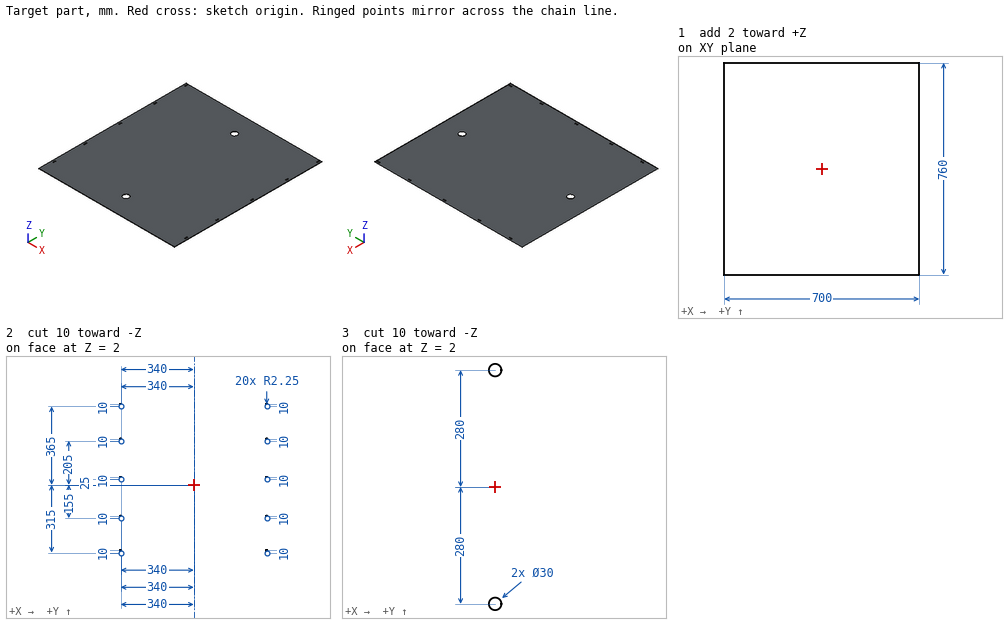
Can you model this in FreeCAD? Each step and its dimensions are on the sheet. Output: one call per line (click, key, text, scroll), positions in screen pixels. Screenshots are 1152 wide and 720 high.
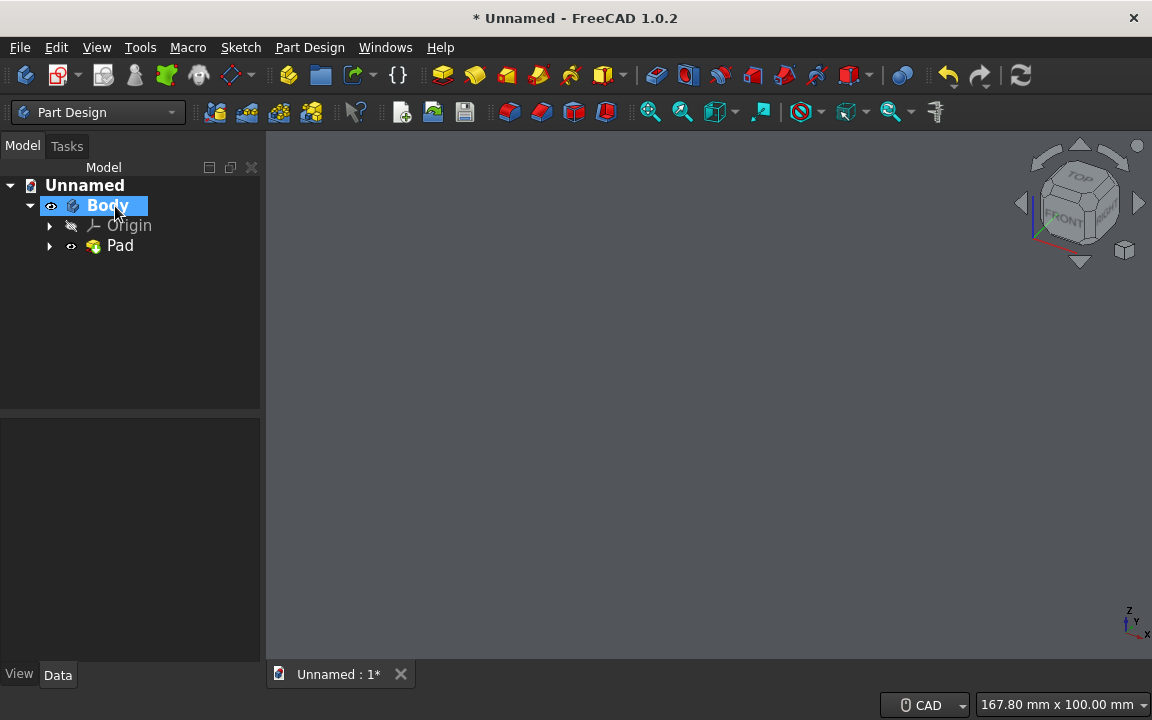
click(652, 112)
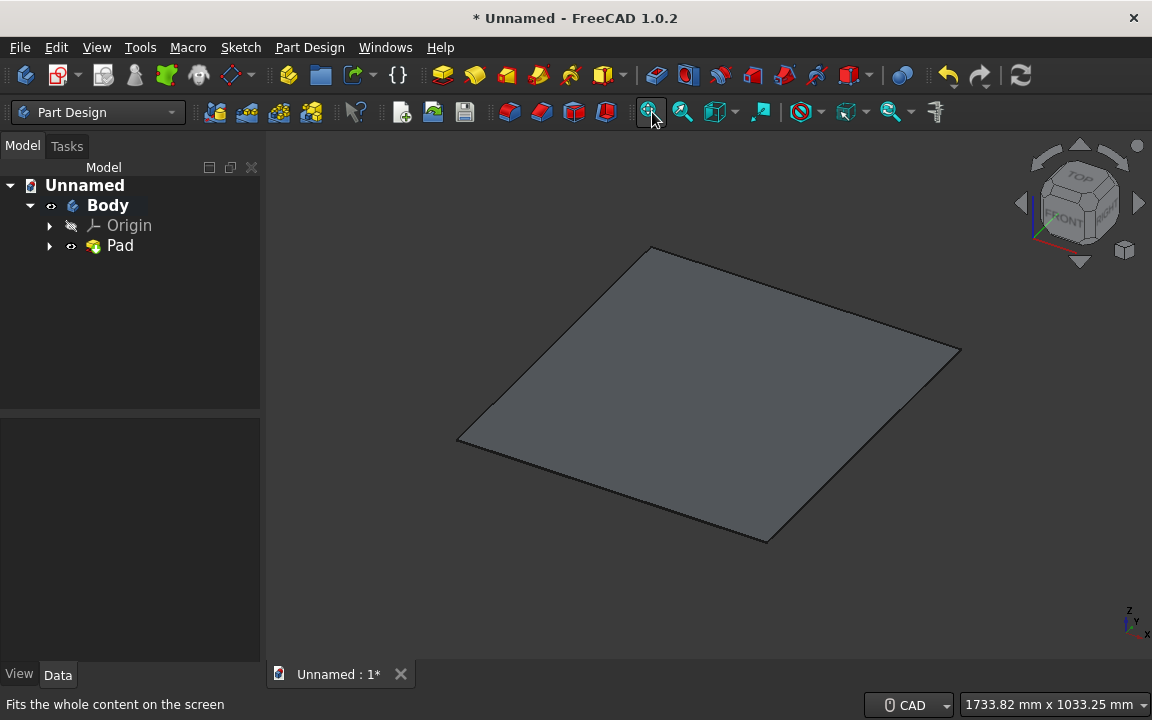
click(709, 394)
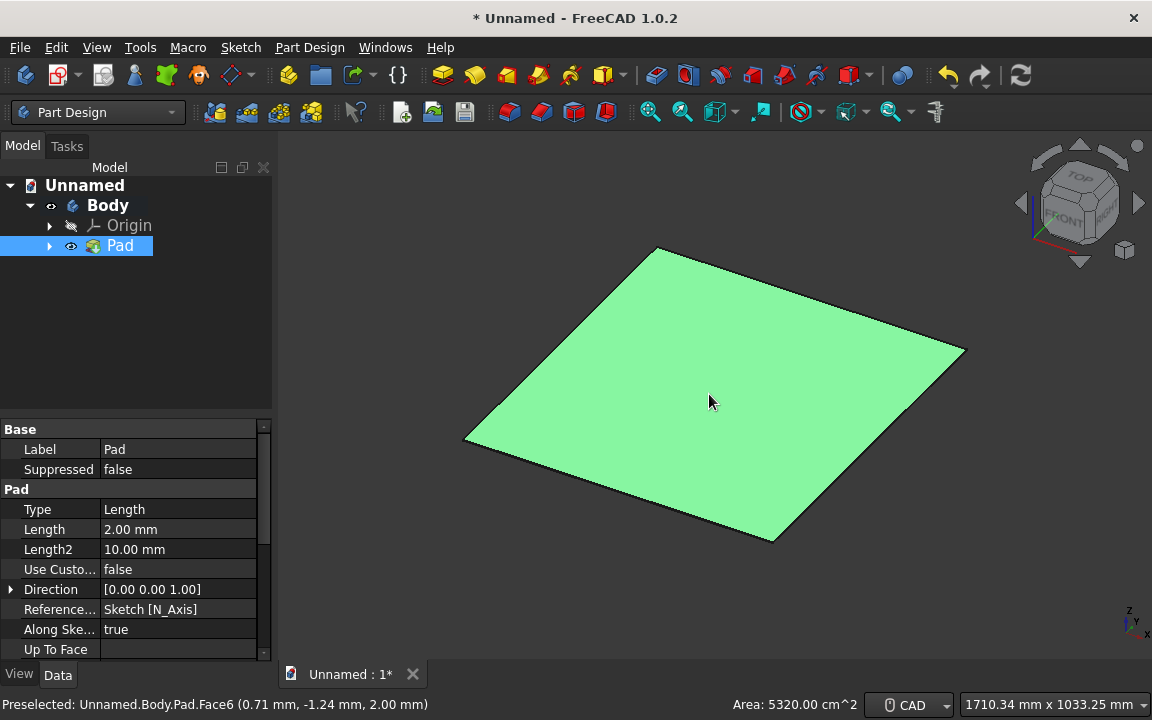
click(58, 76)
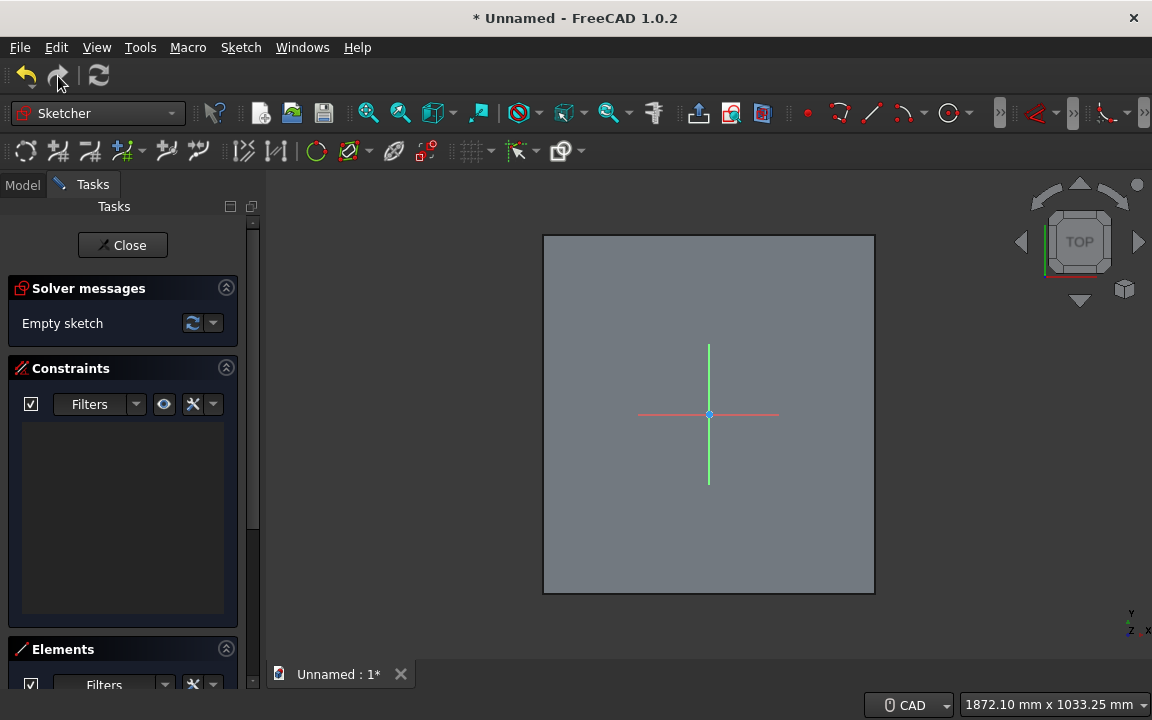
key(g)
key(s)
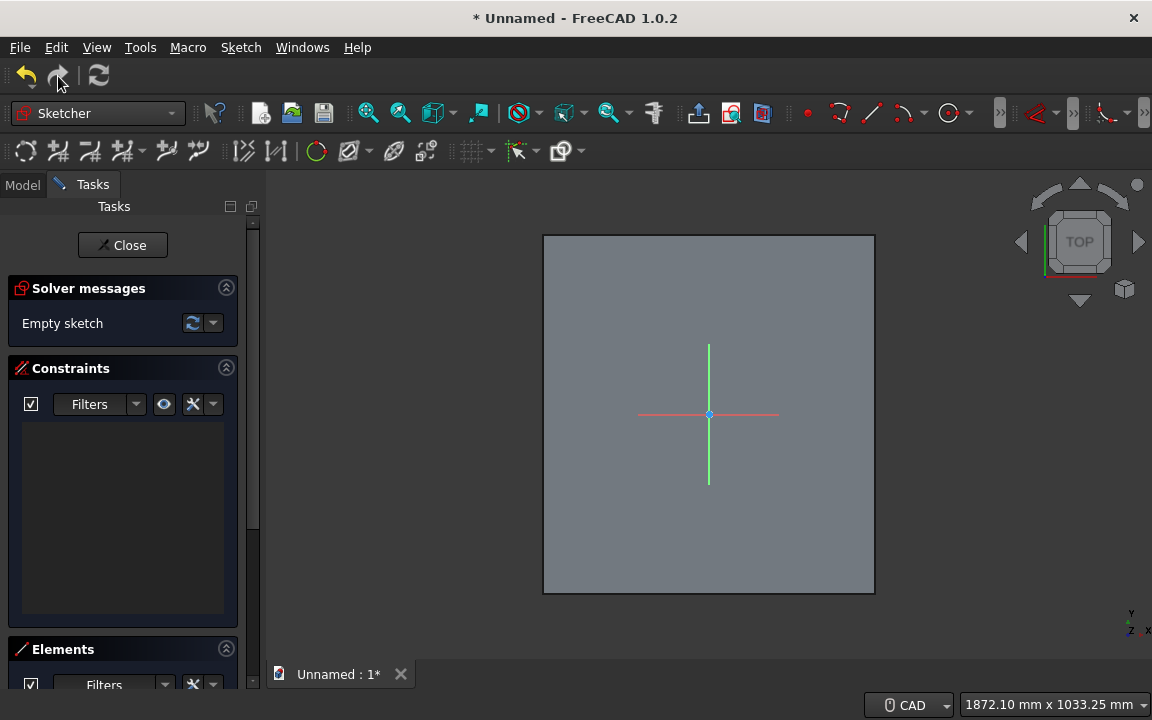
scroll(548, 242, up, 16)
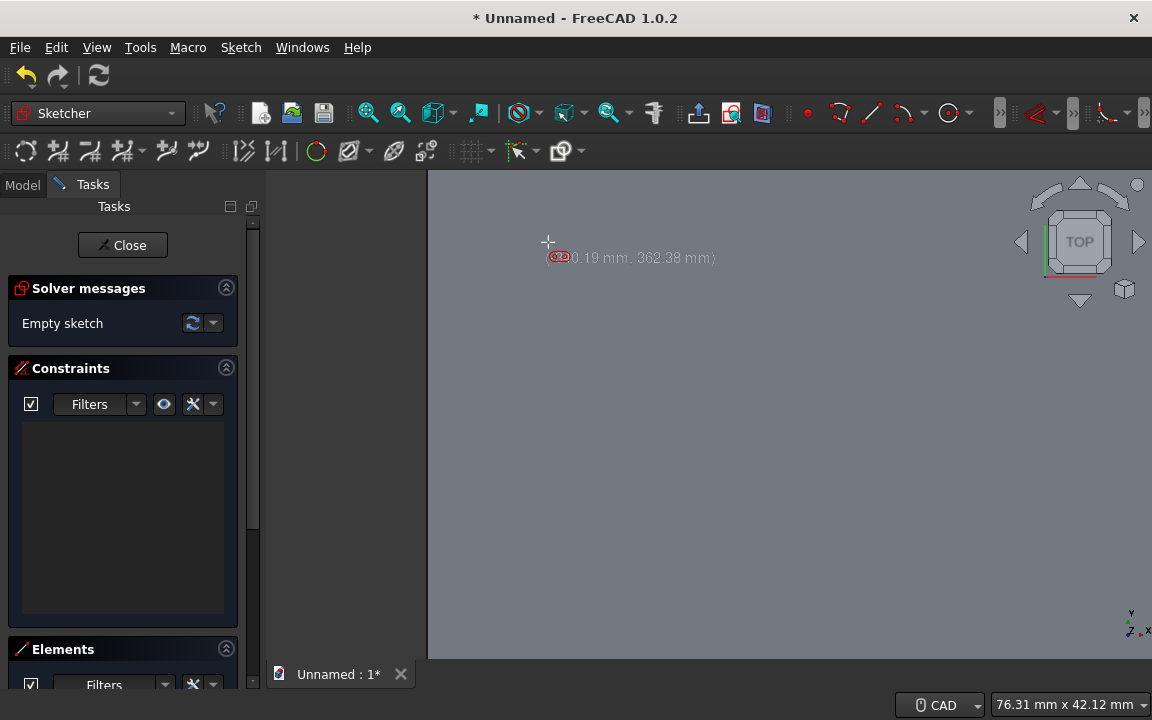
scroll(477, 257, down, 16)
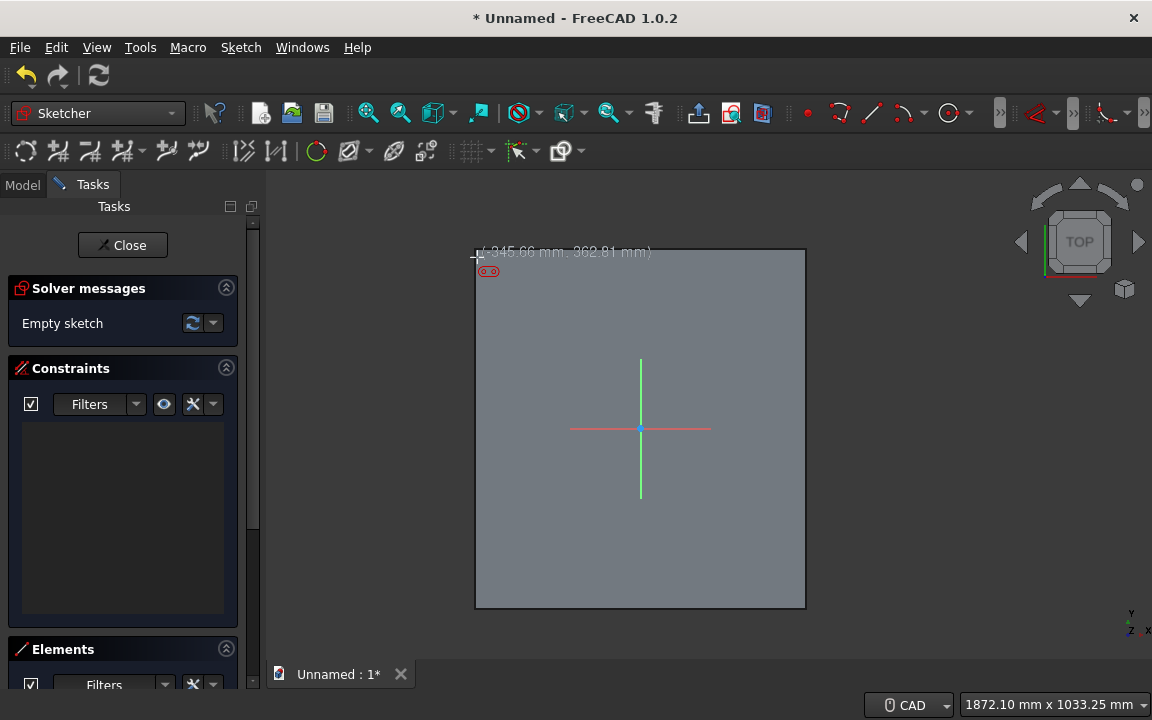
click(480, 256)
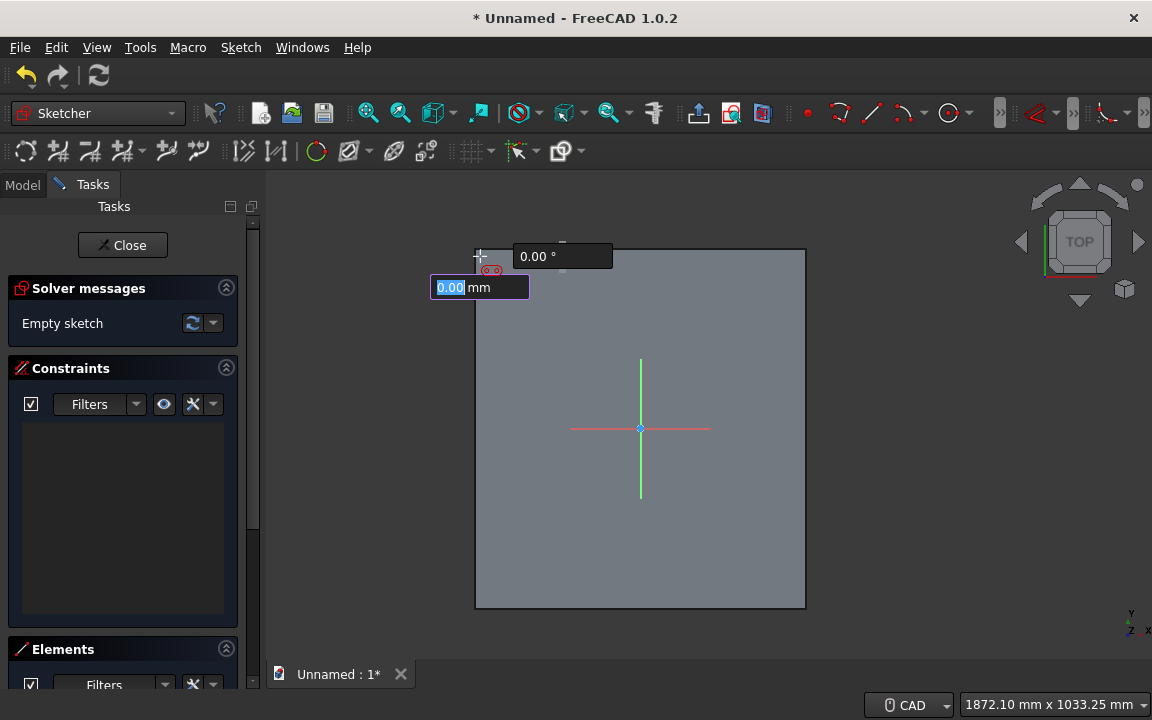
scroll(480, 251, up, 7)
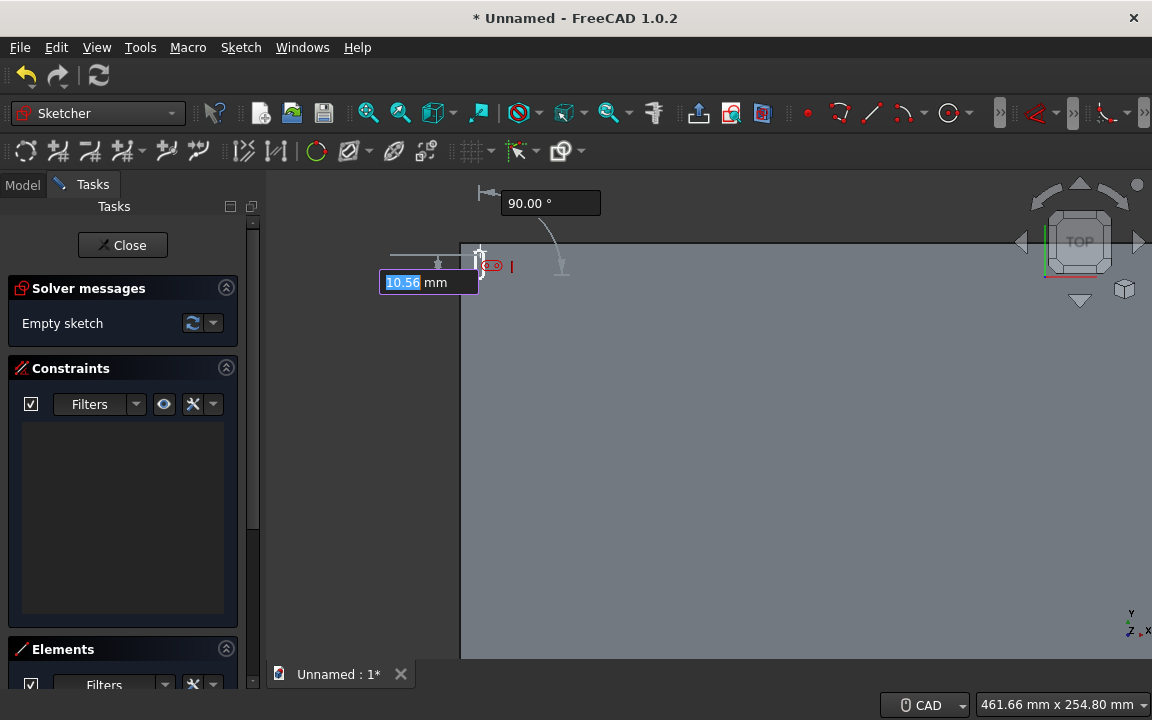
click(479, 252)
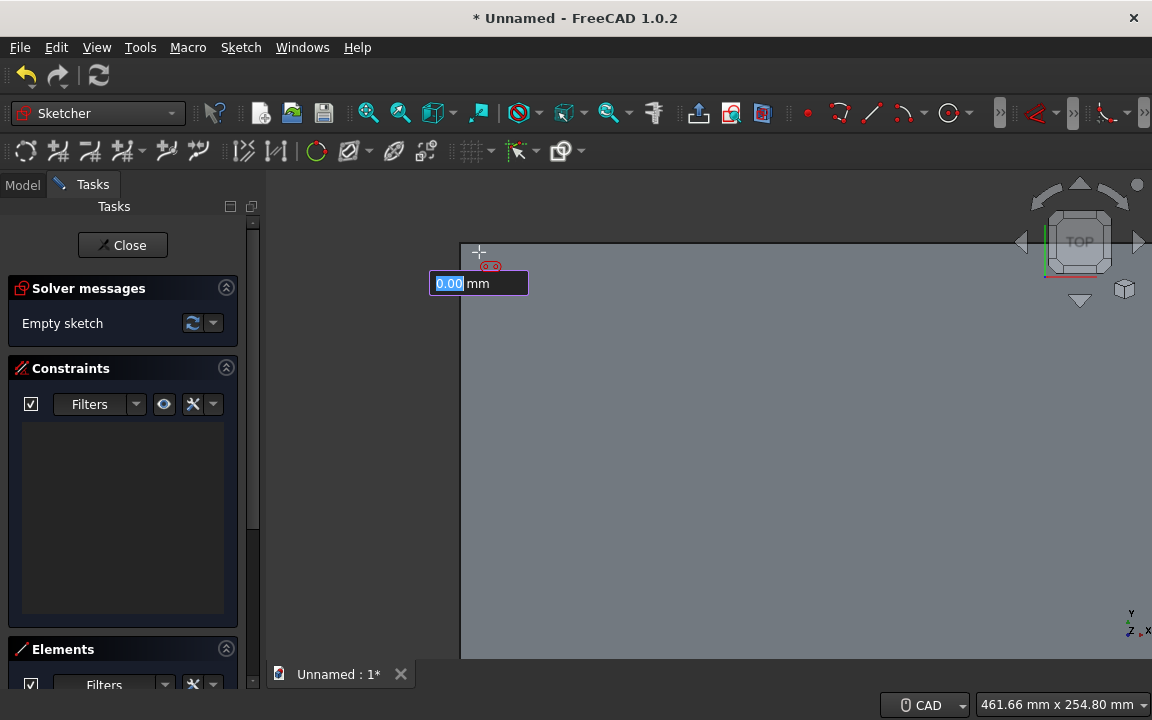
scroll(483, 262, up, 7)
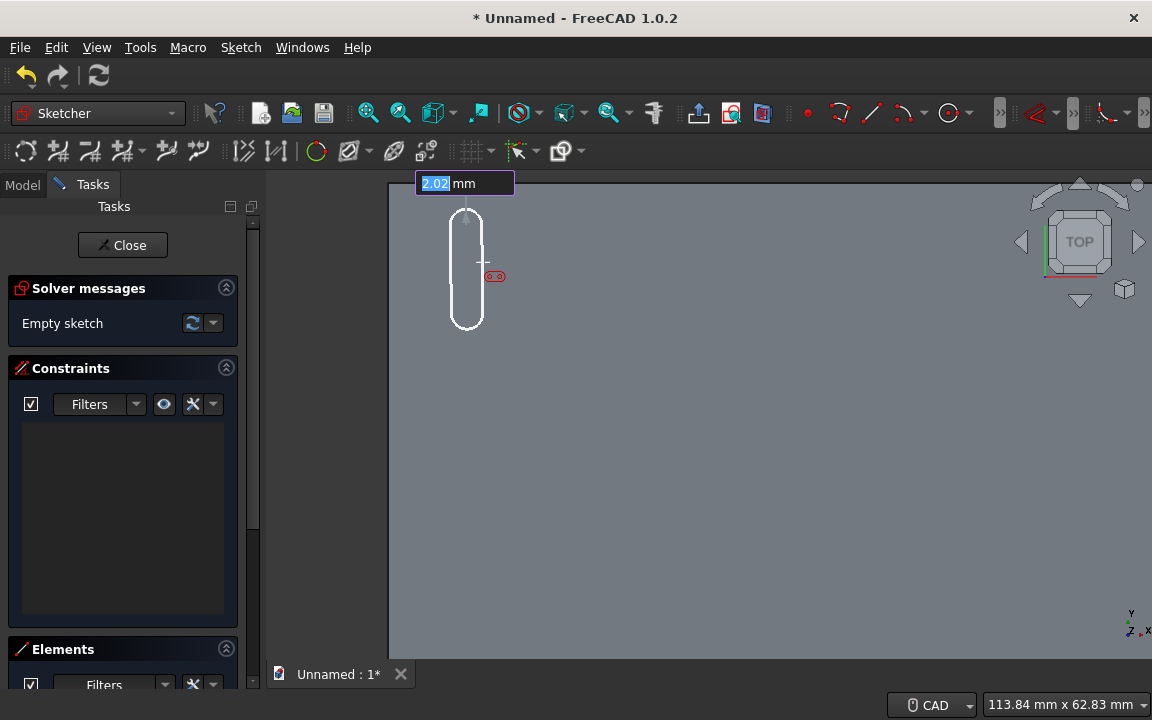
click(483, 261)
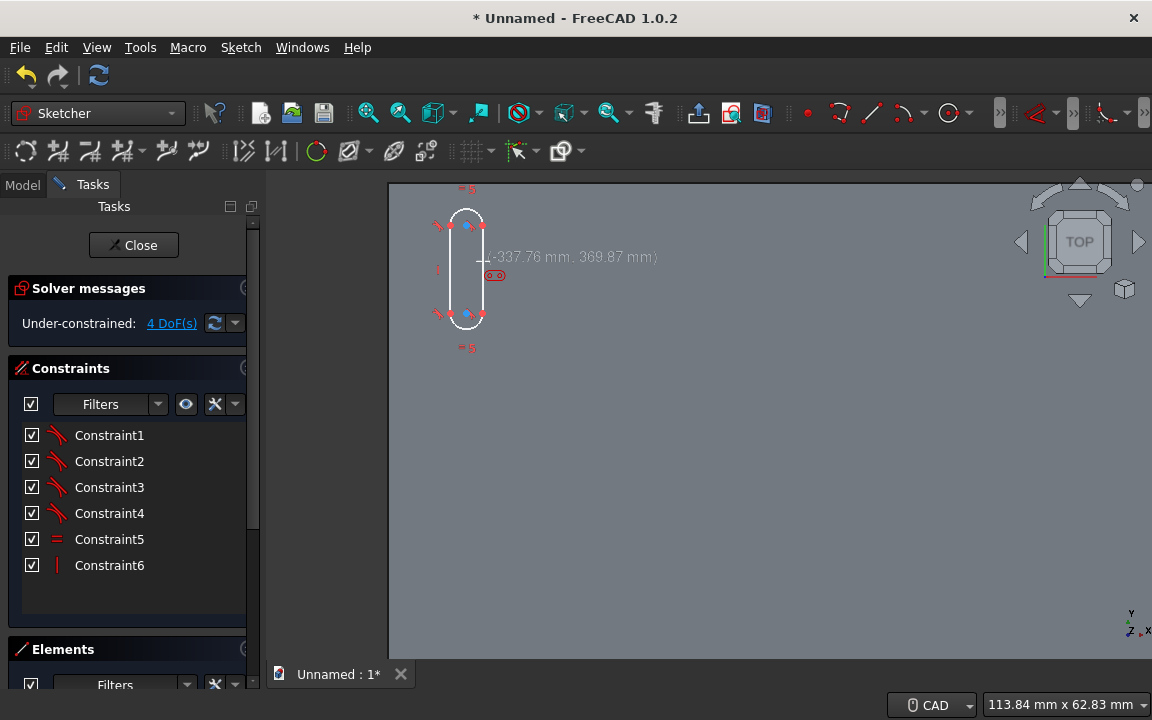
scroll(480, 253, down, 14)